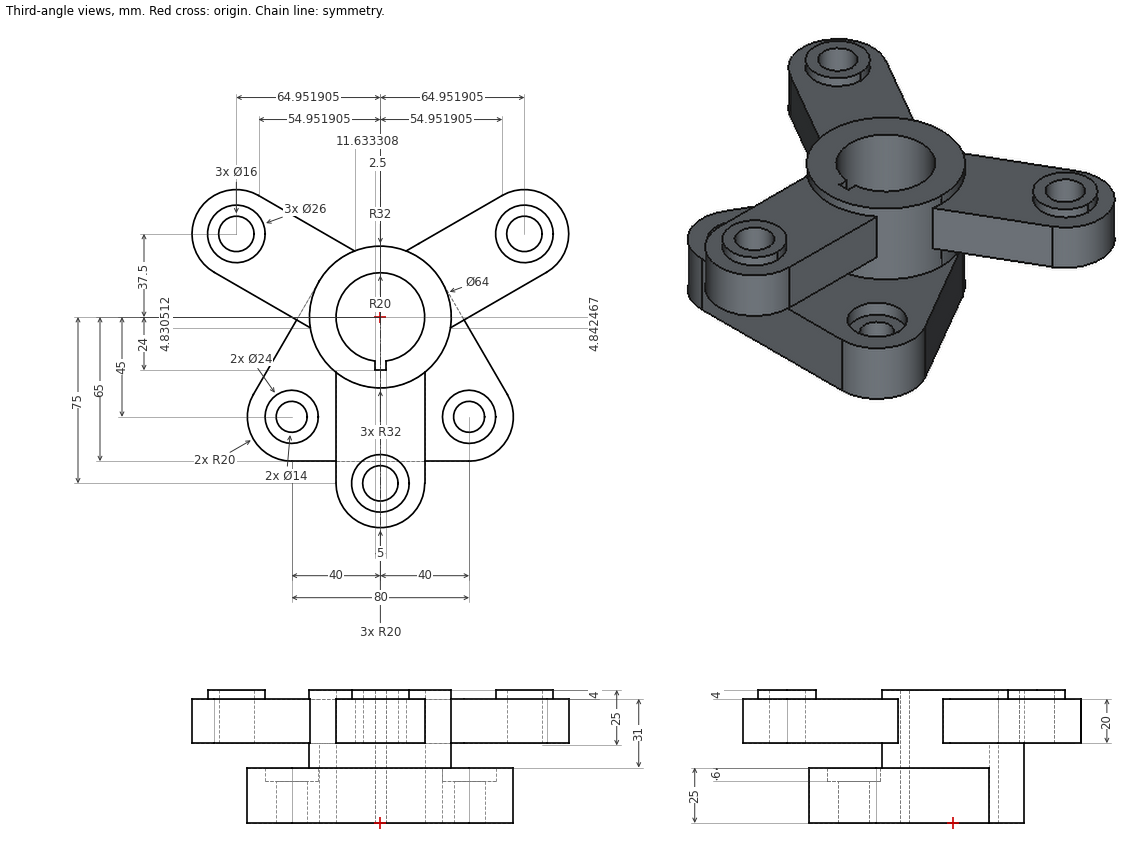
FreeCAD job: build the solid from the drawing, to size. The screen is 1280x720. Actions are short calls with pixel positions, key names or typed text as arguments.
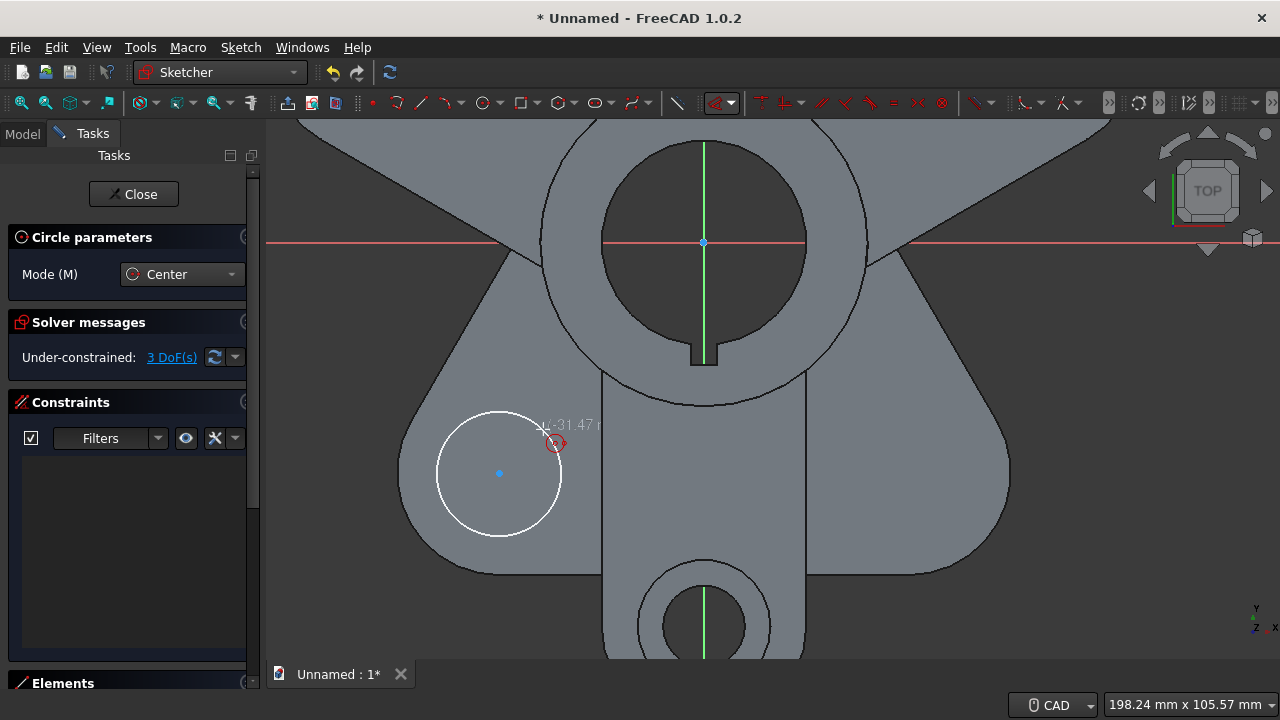
click(909, 473)
click(952, 429)
key(Escape)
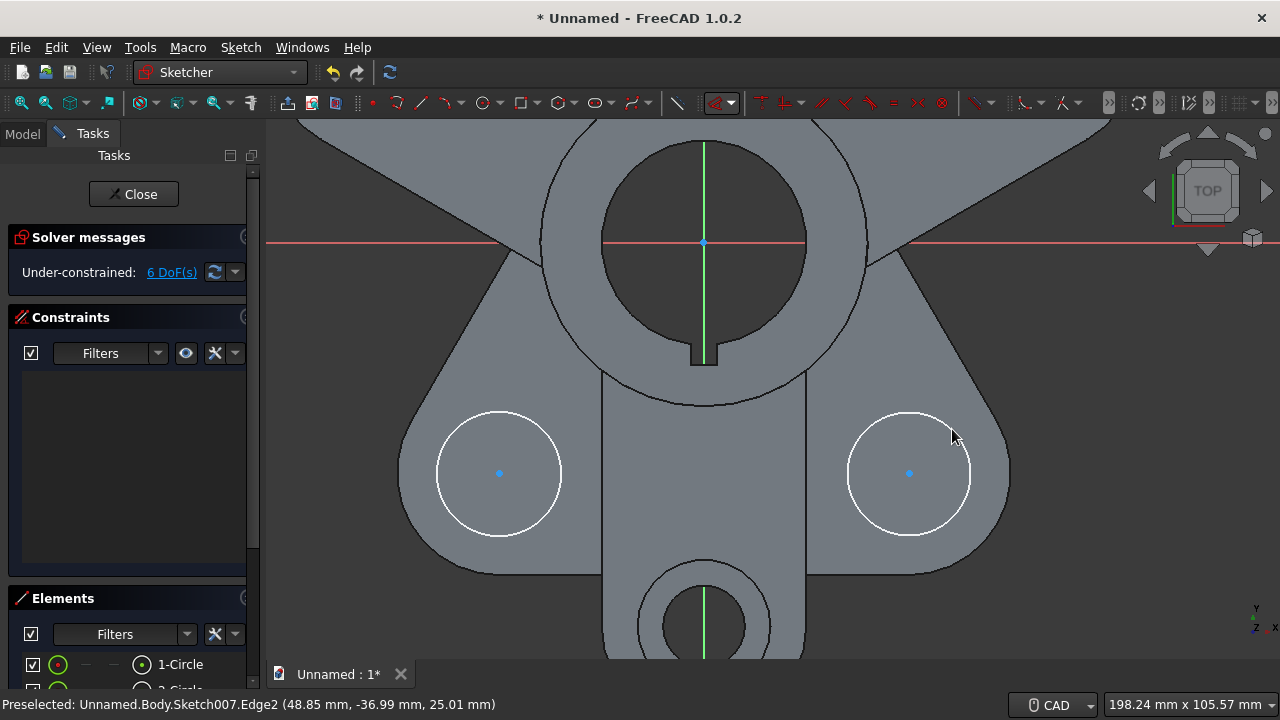
click(543, 430)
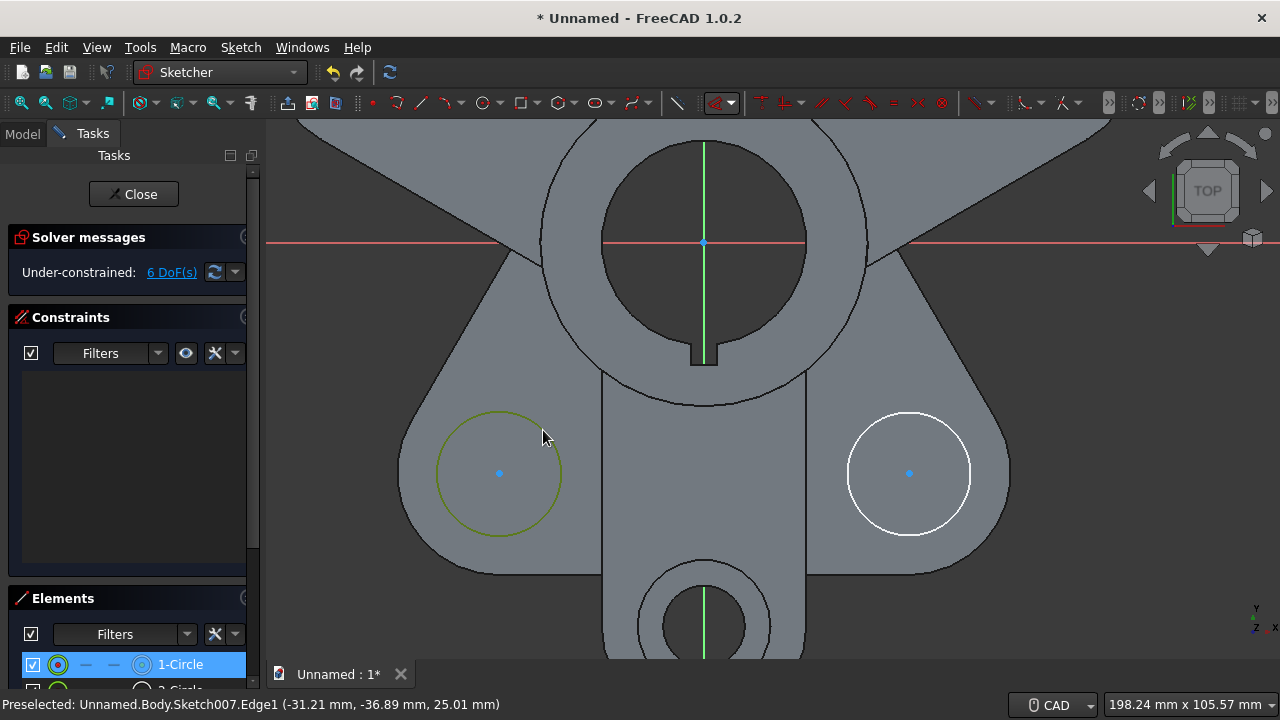
click(952, 430)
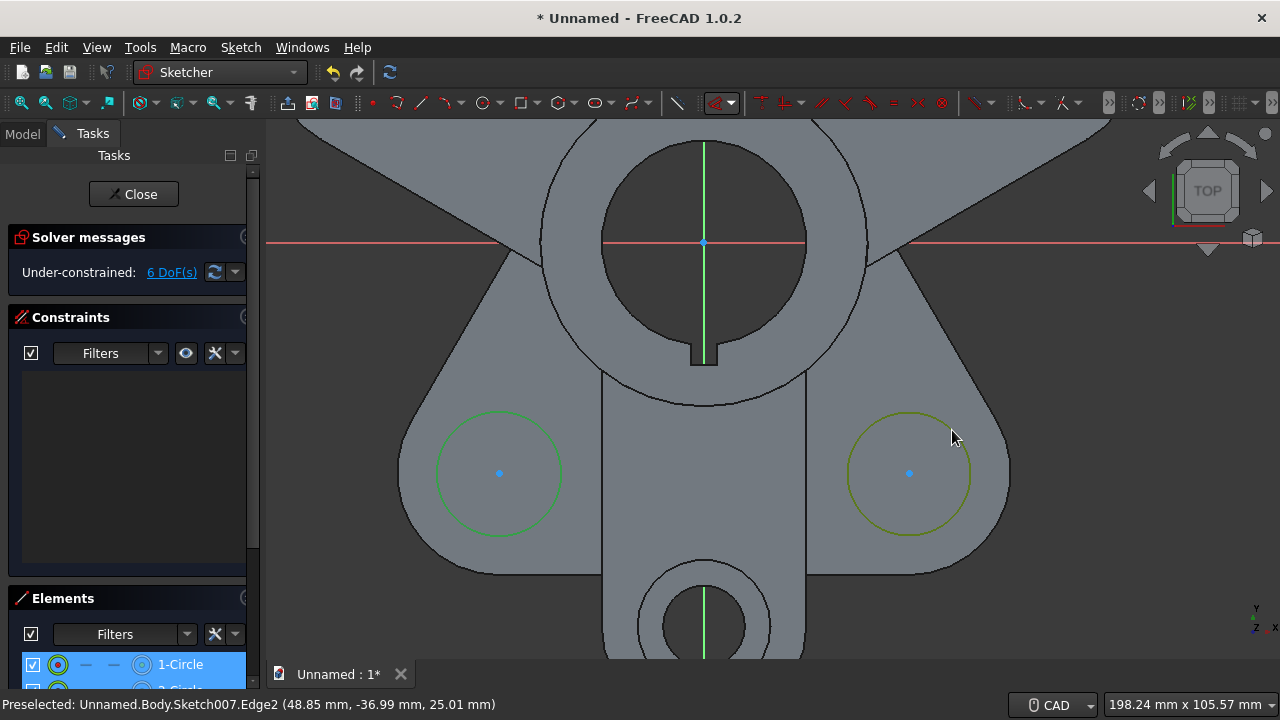
key(e)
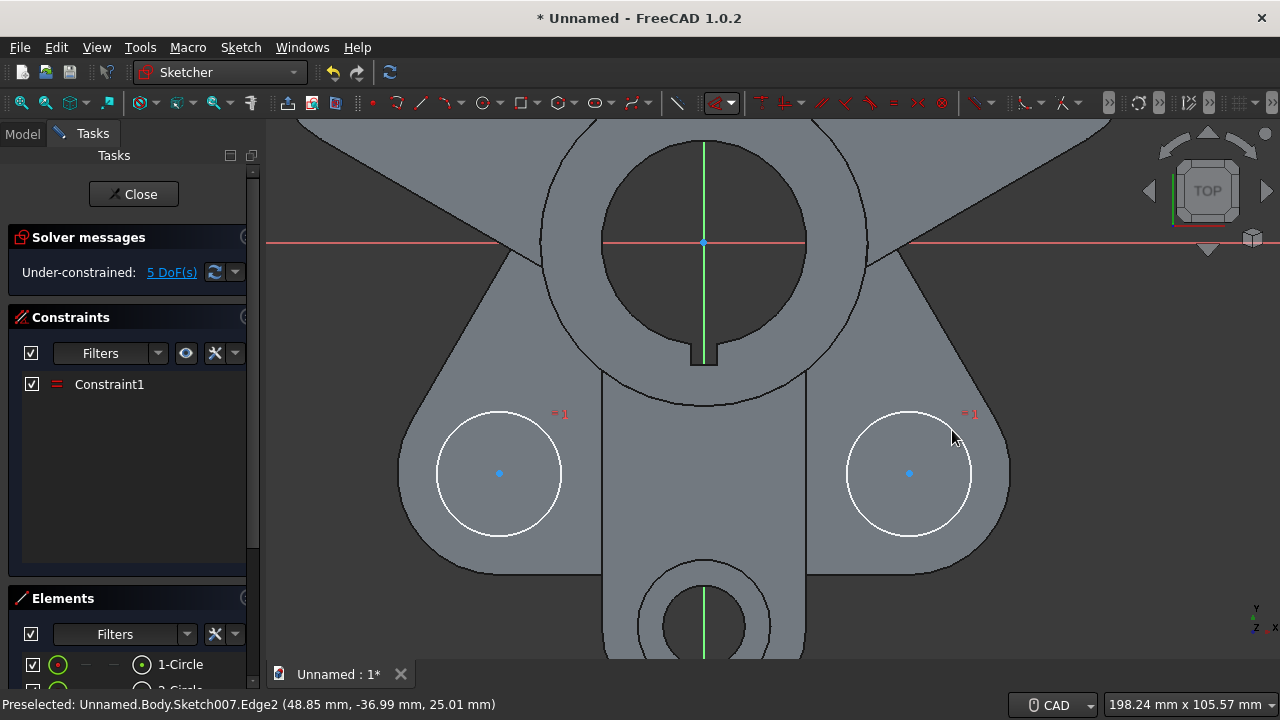
click(499, 474)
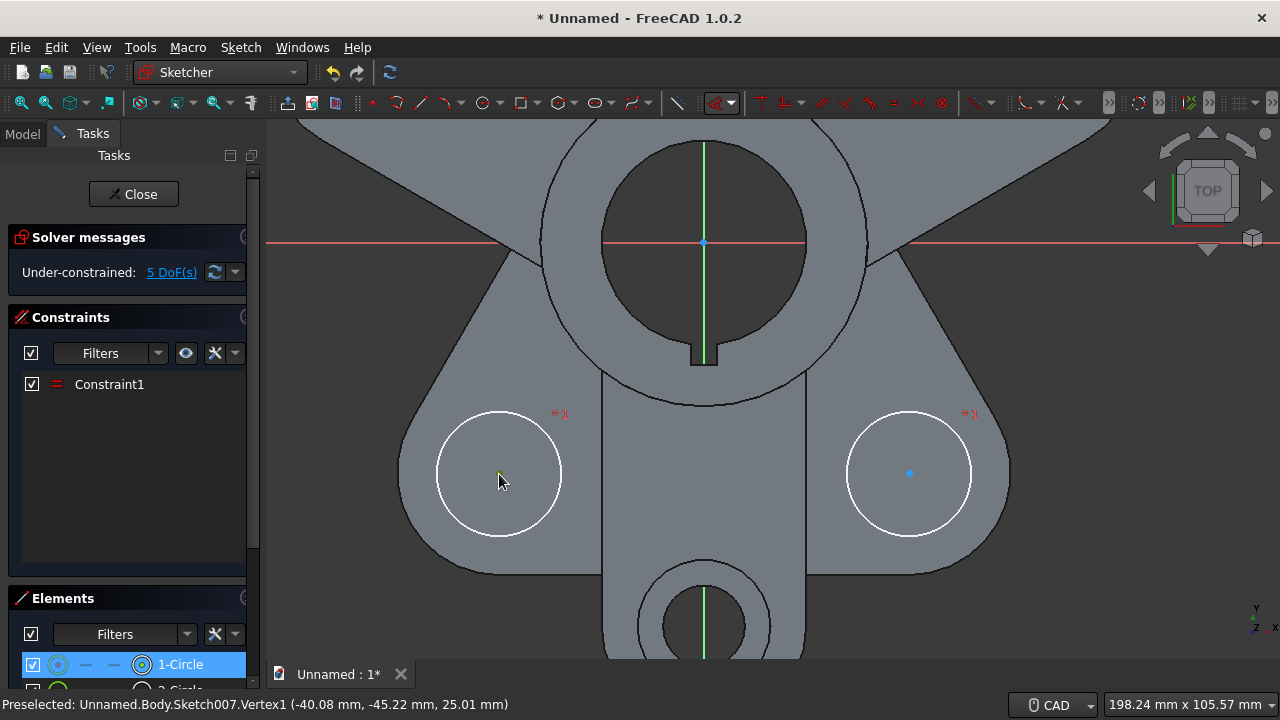
click(909, 474)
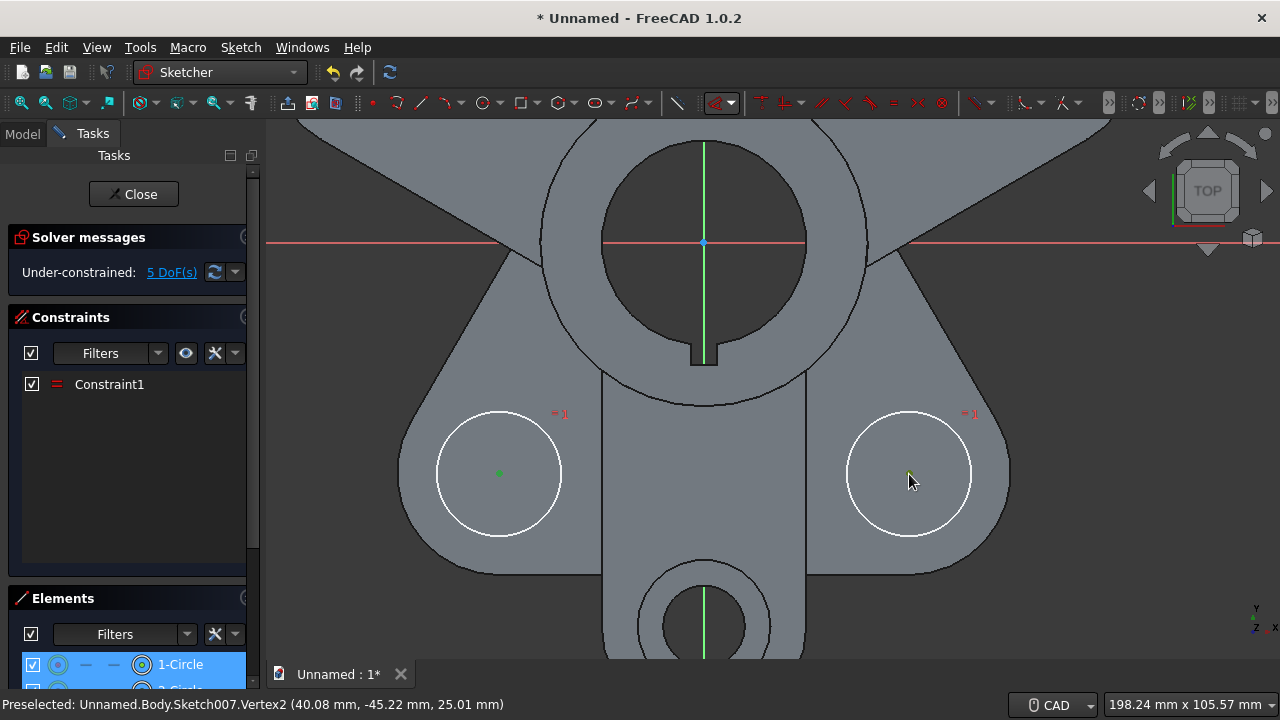
key(h)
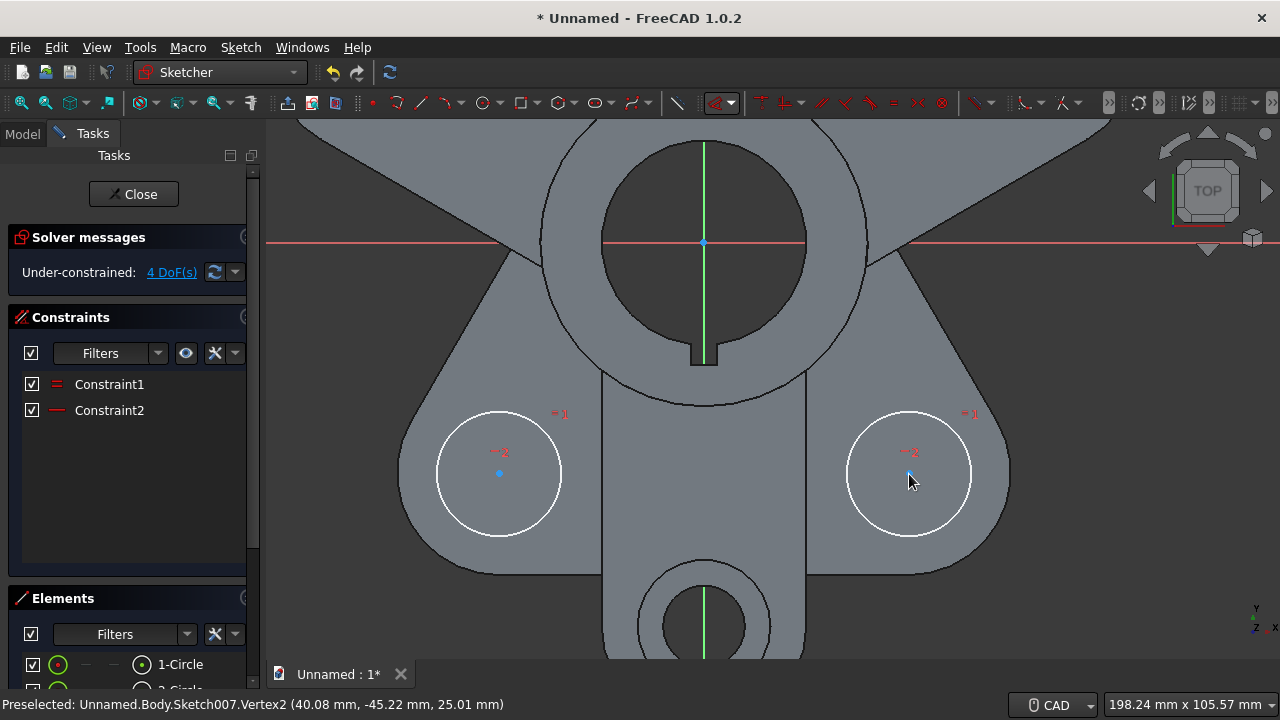
click(543, 430)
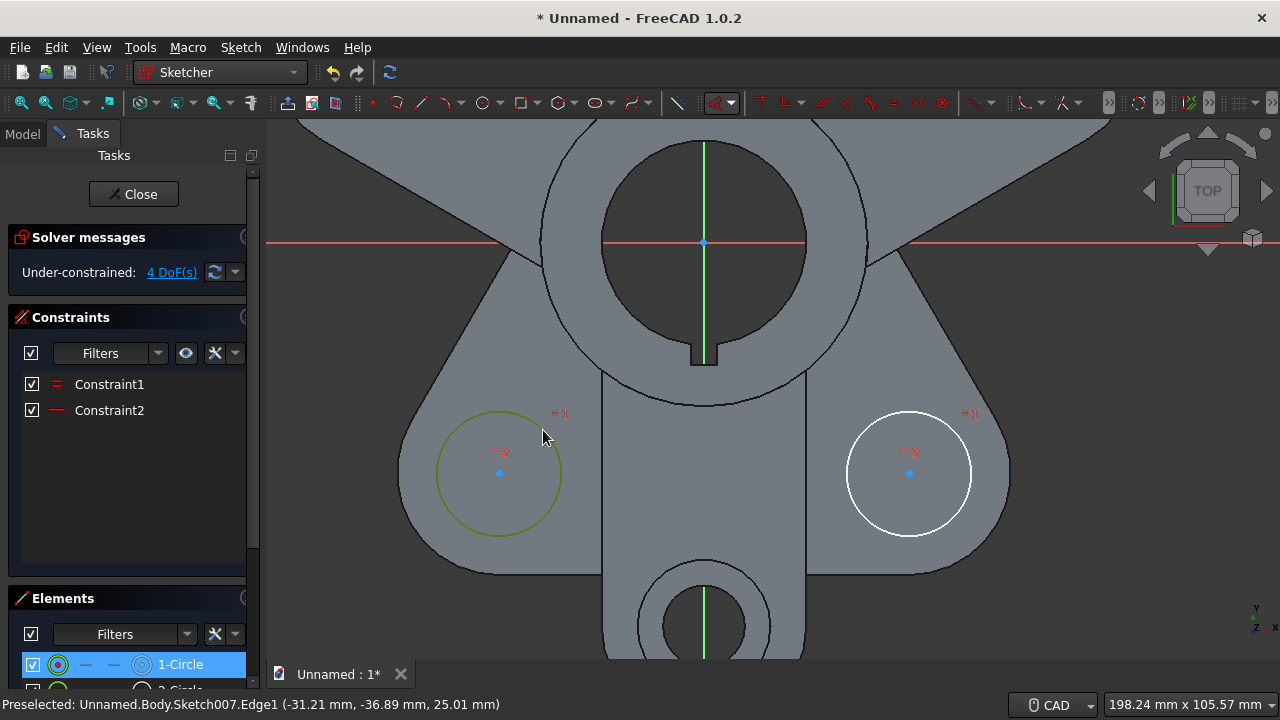
click(734, 104)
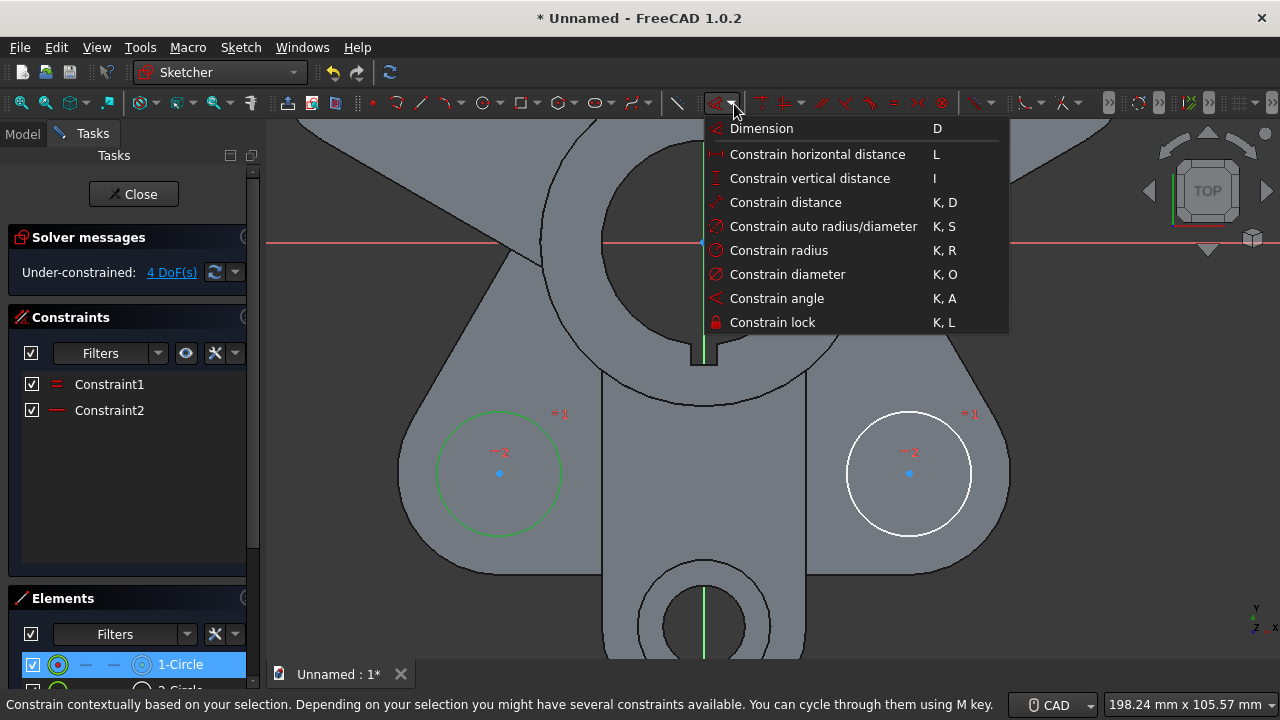
click(857, 274)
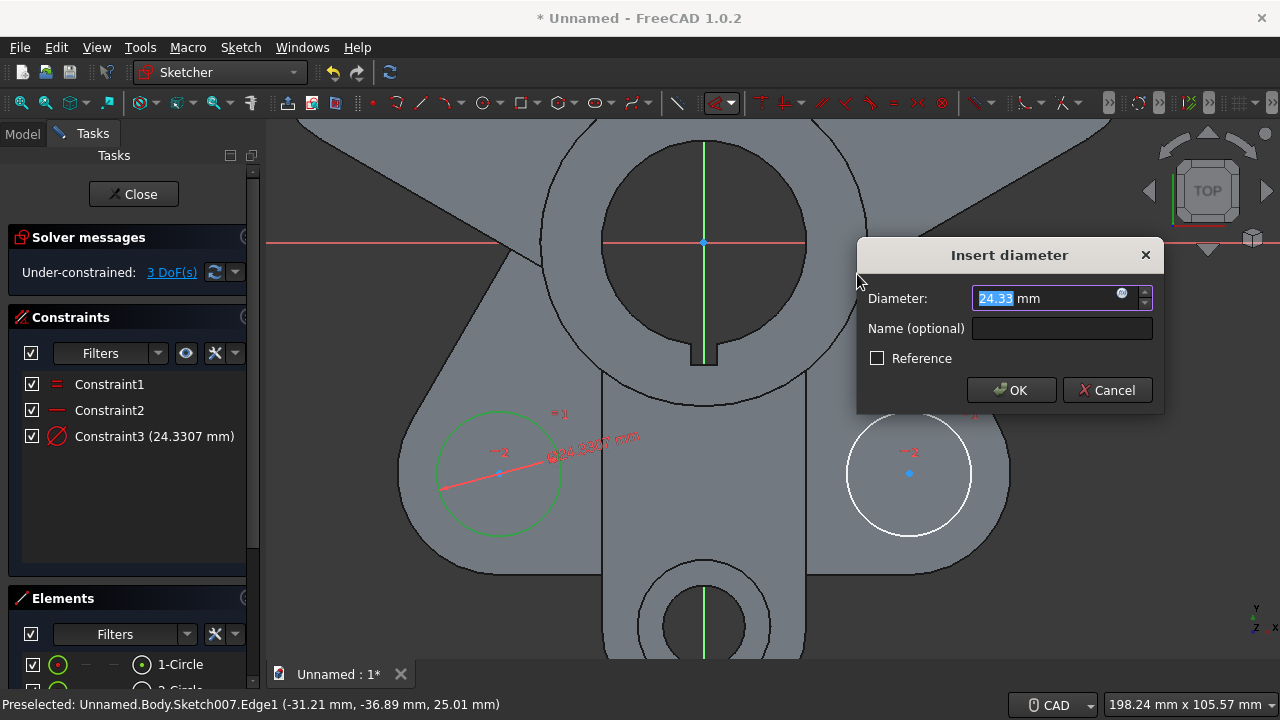
text(24)
key(Return)